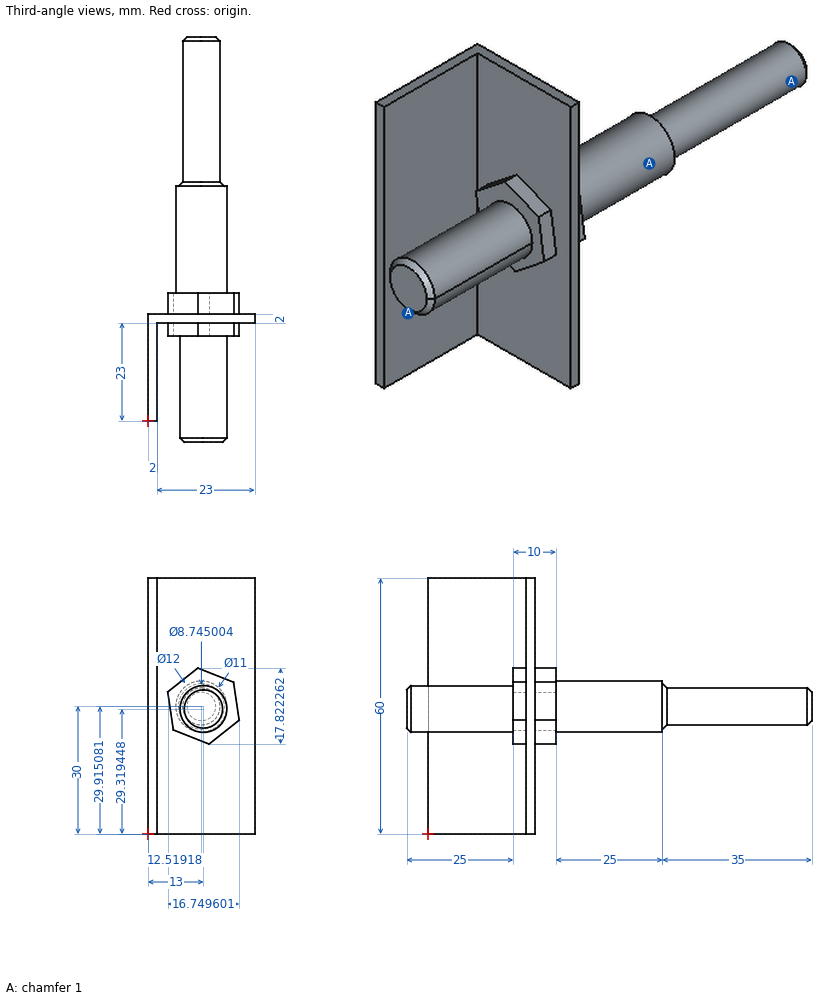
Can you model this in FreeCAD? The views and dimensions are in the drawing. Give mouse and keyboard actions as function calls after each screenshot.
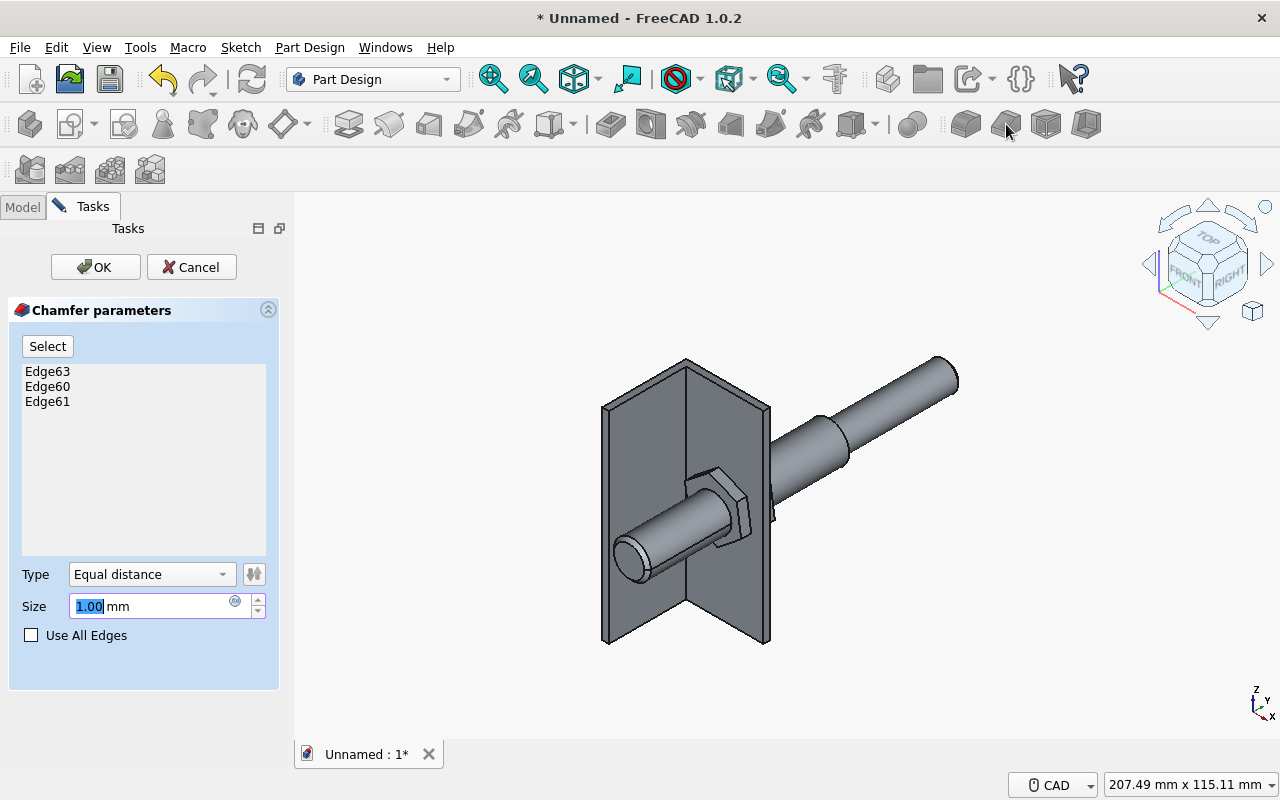
text(1)
key(Tab)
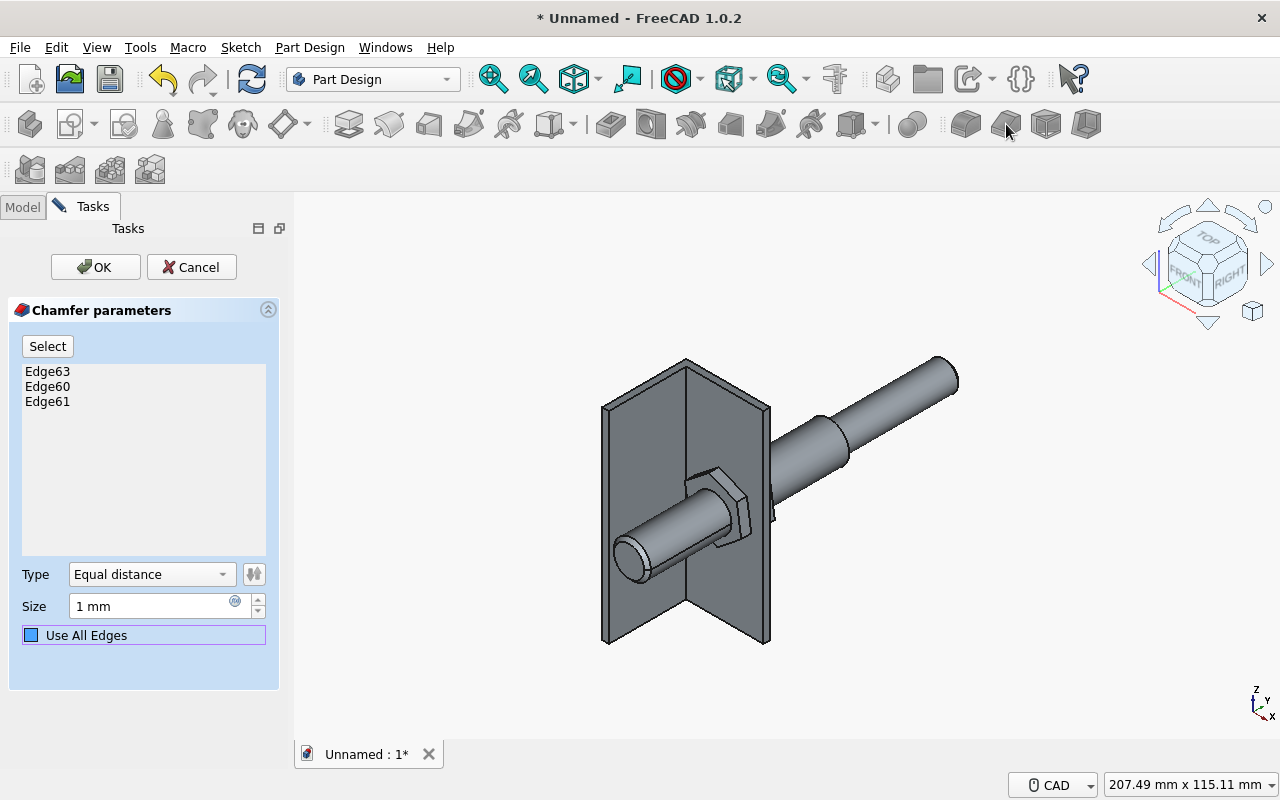
click(96, 267)